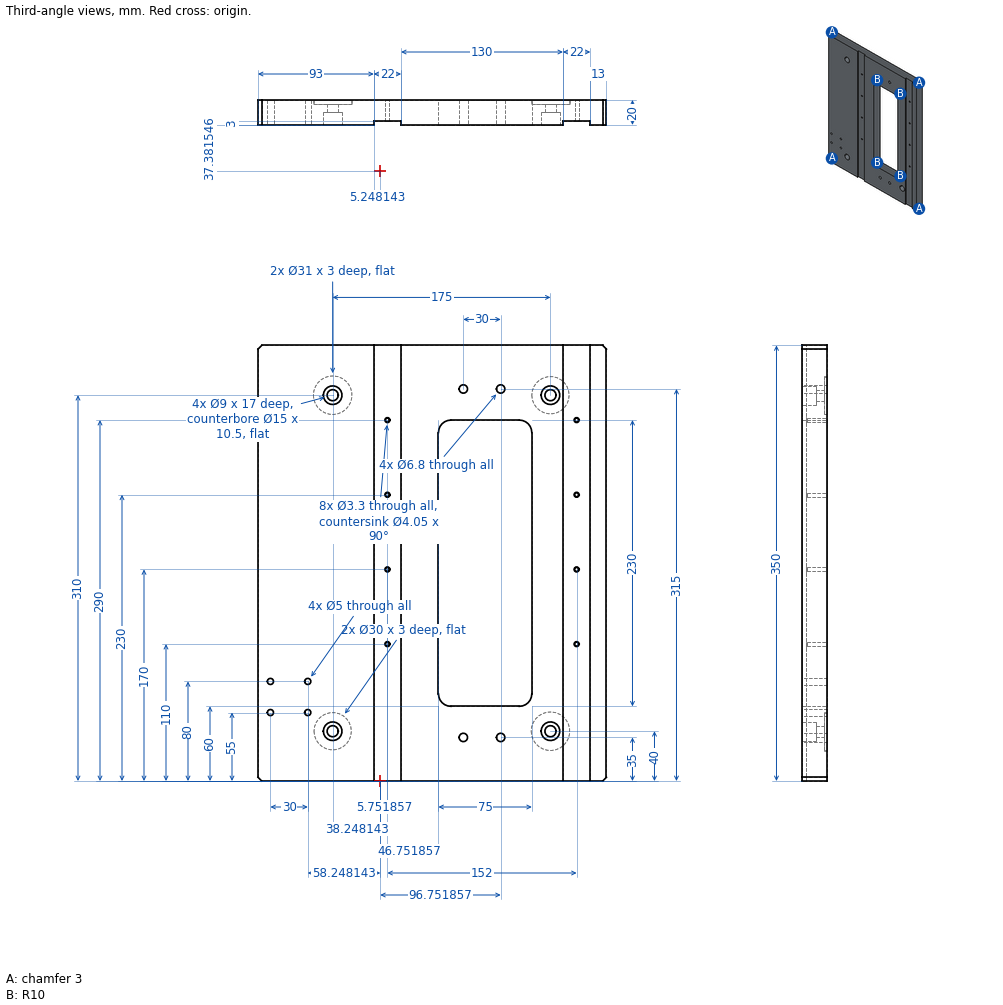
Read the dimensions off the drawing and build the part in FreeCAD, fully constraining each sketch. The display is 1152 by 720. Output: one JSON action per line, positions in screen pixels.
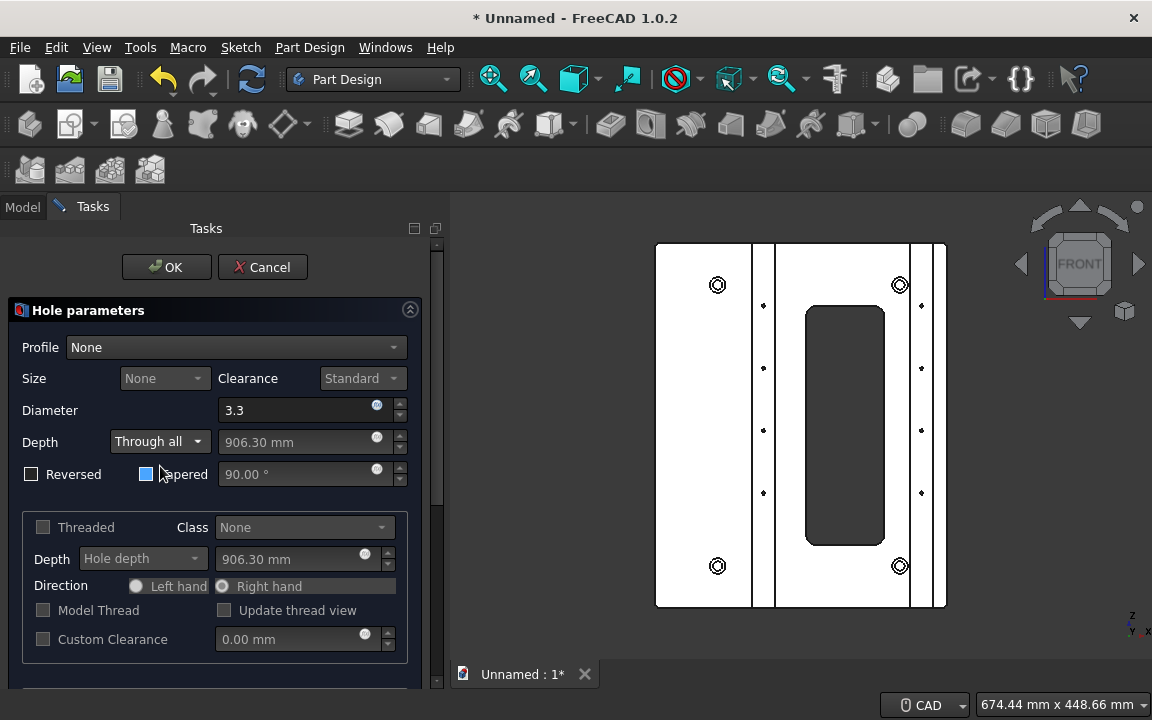
{"action": "scroll", "coordinate": [437, 463], "scroll_direction": "down", "scroll_amount": 2}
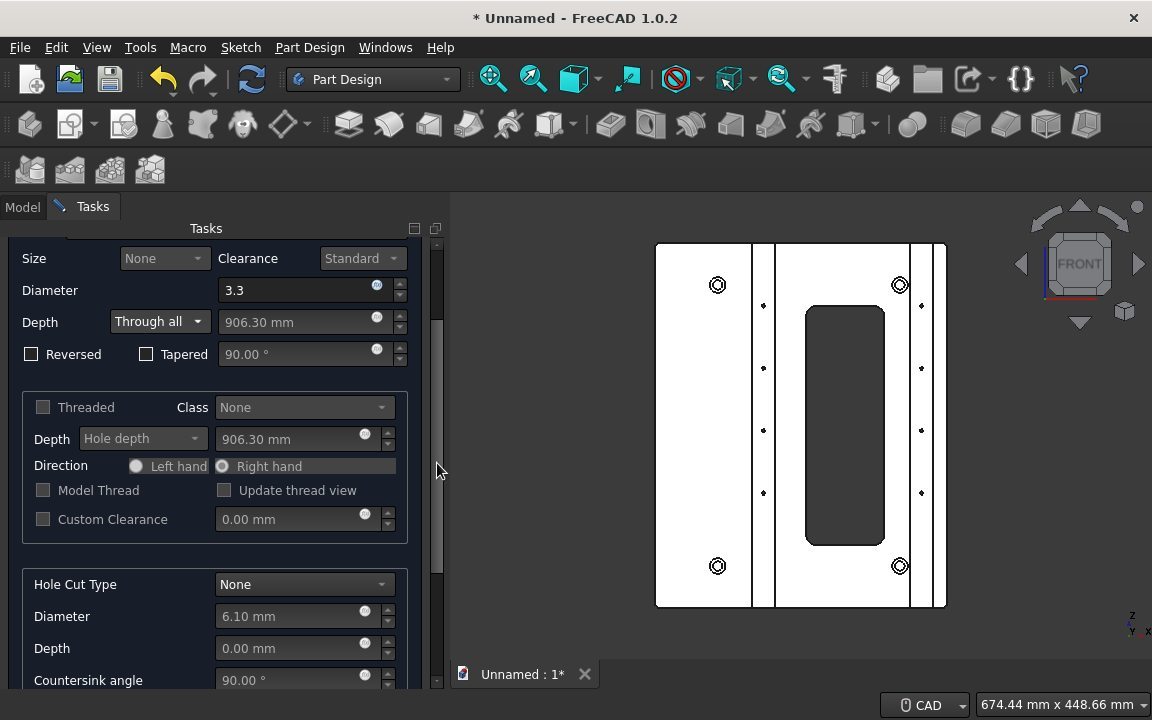
{"action": "left_click", "coordinate": [306, 584]}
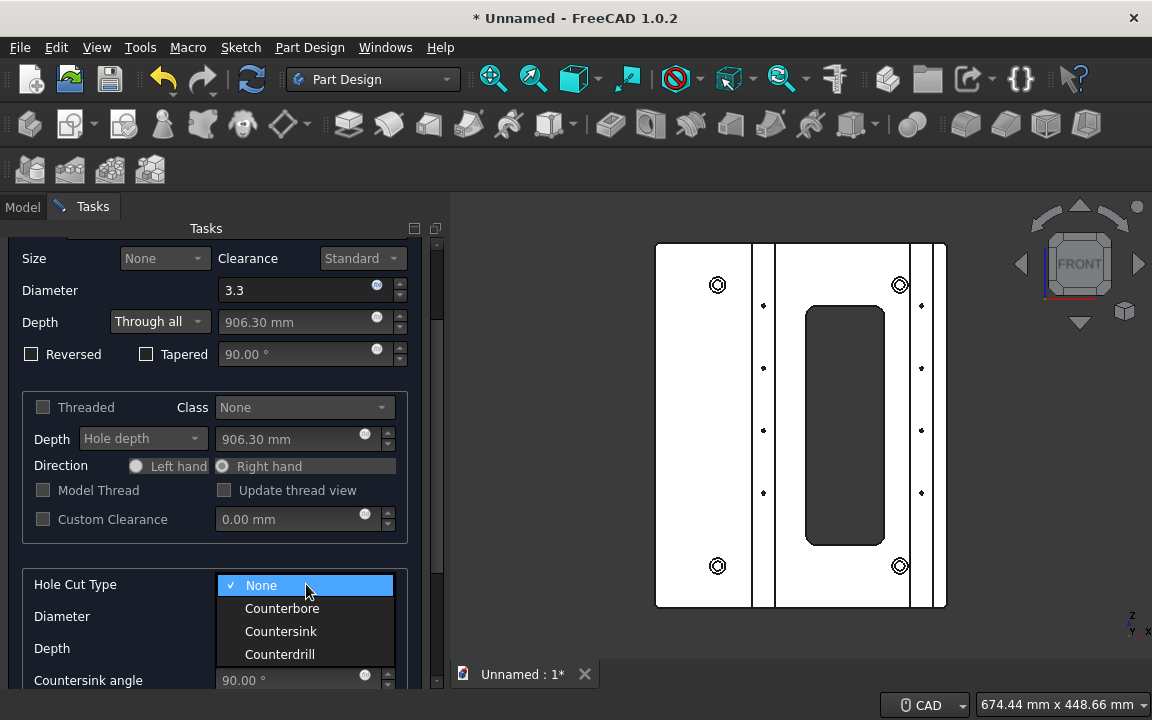
{"action": "left_click", "coordinate": [304, 632]}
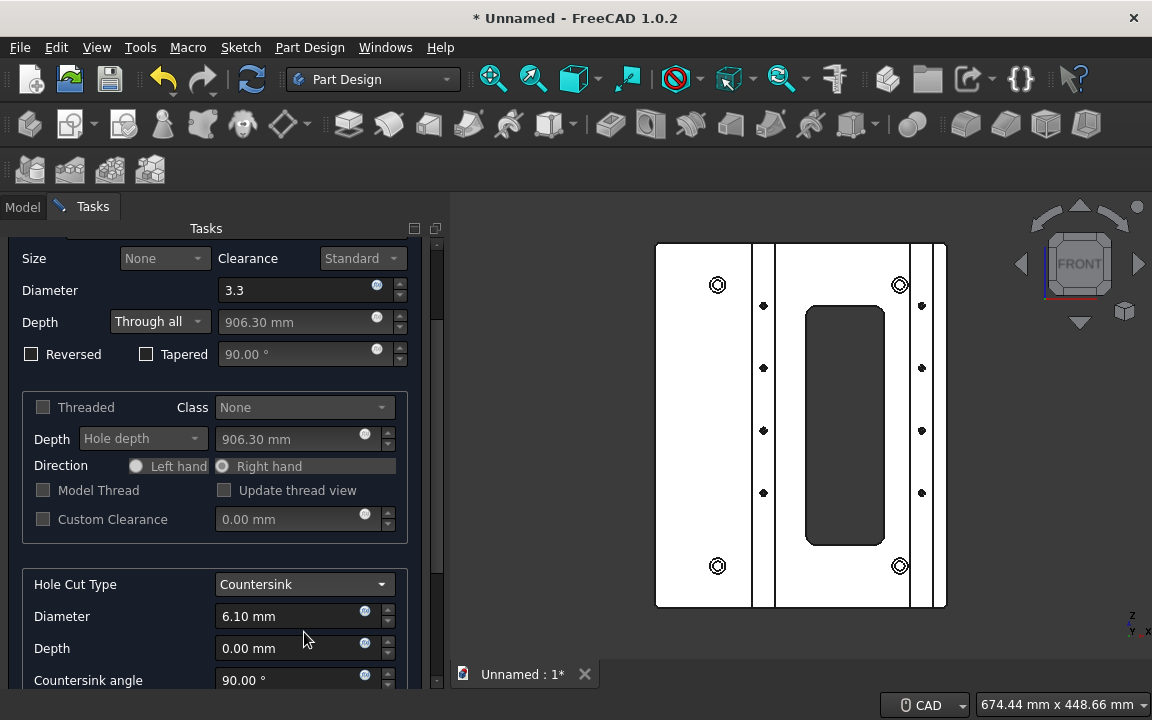
{"action": "triple_click", "coordinate": [298, 616]}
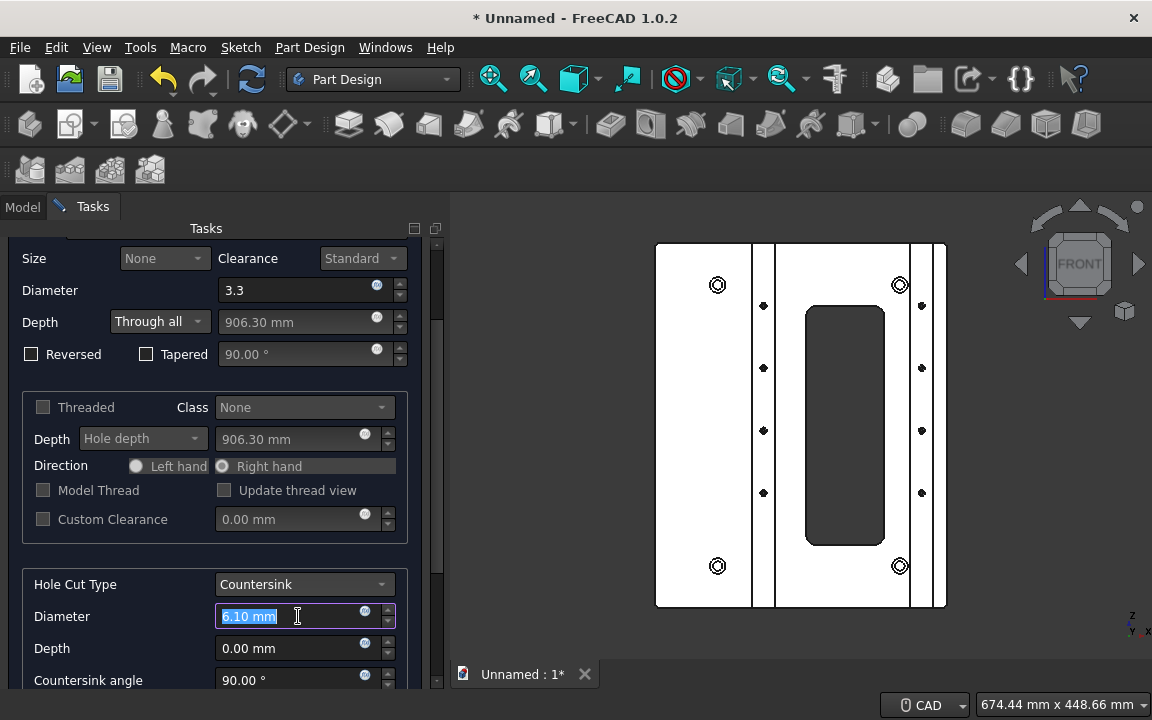
{"action": "type", "text": "4.05"}
{"action": "key", "text": "Tab"}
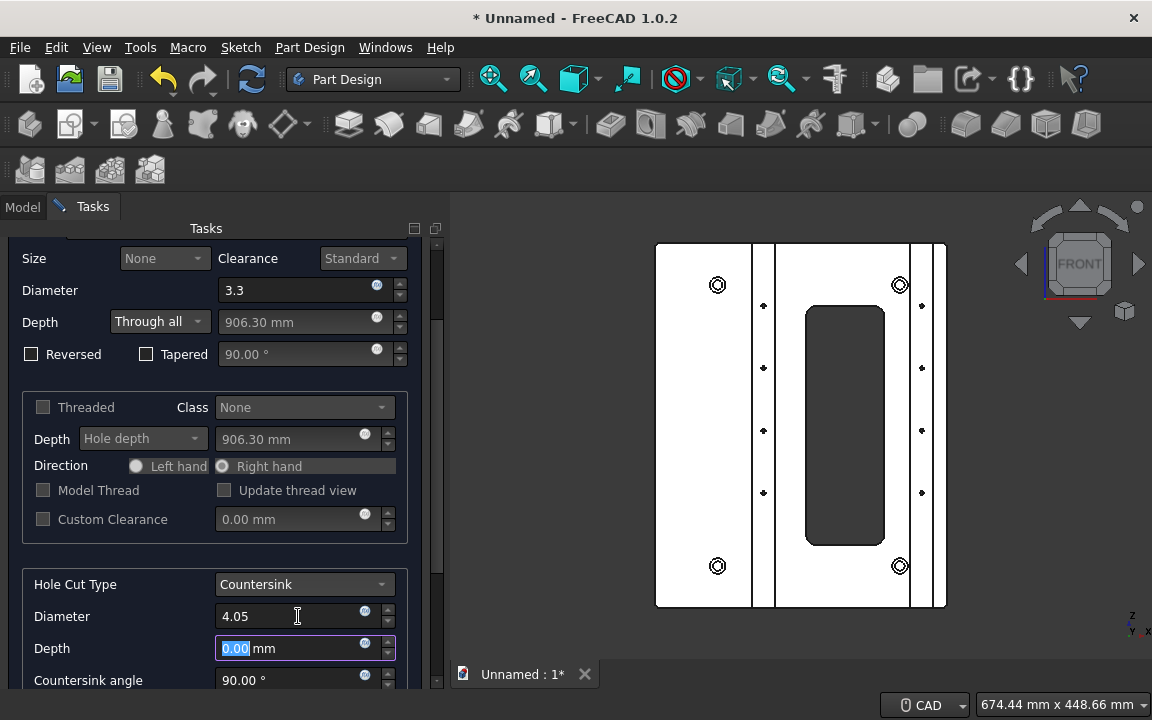
{"action": "scroll", "coordinate": [437, 463], "scroll_direction": "up", "scroll_amount": 3}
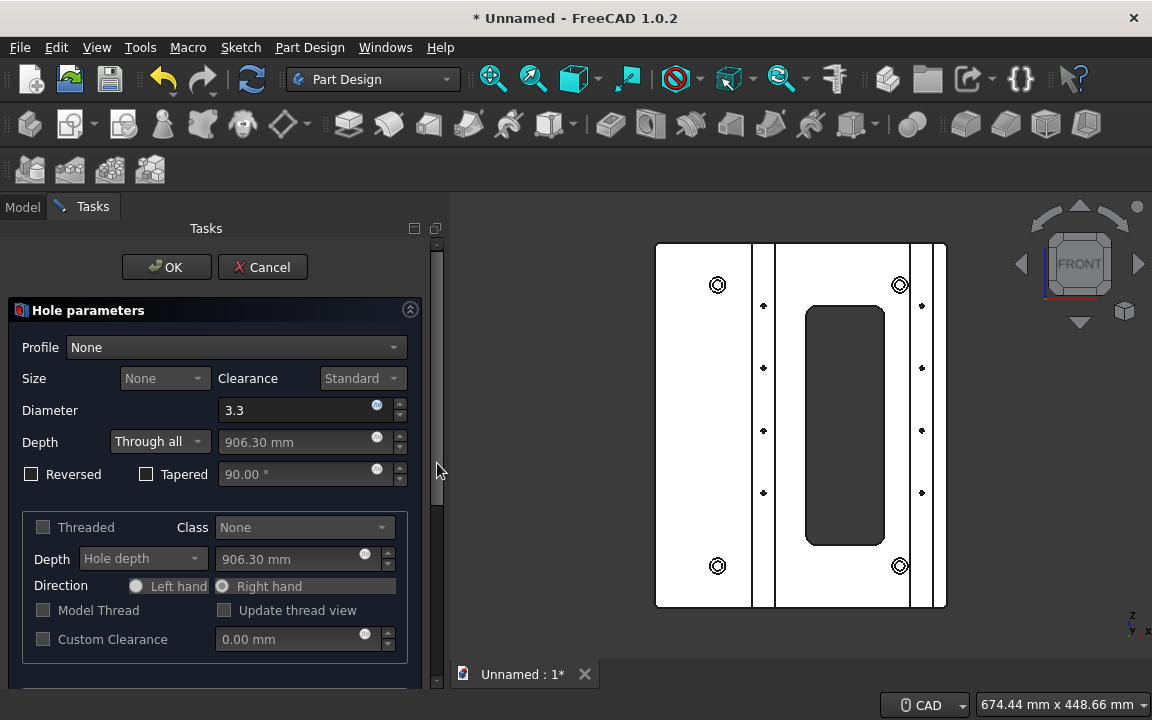
{"action": "left_click", "coordinate": [167, 267]}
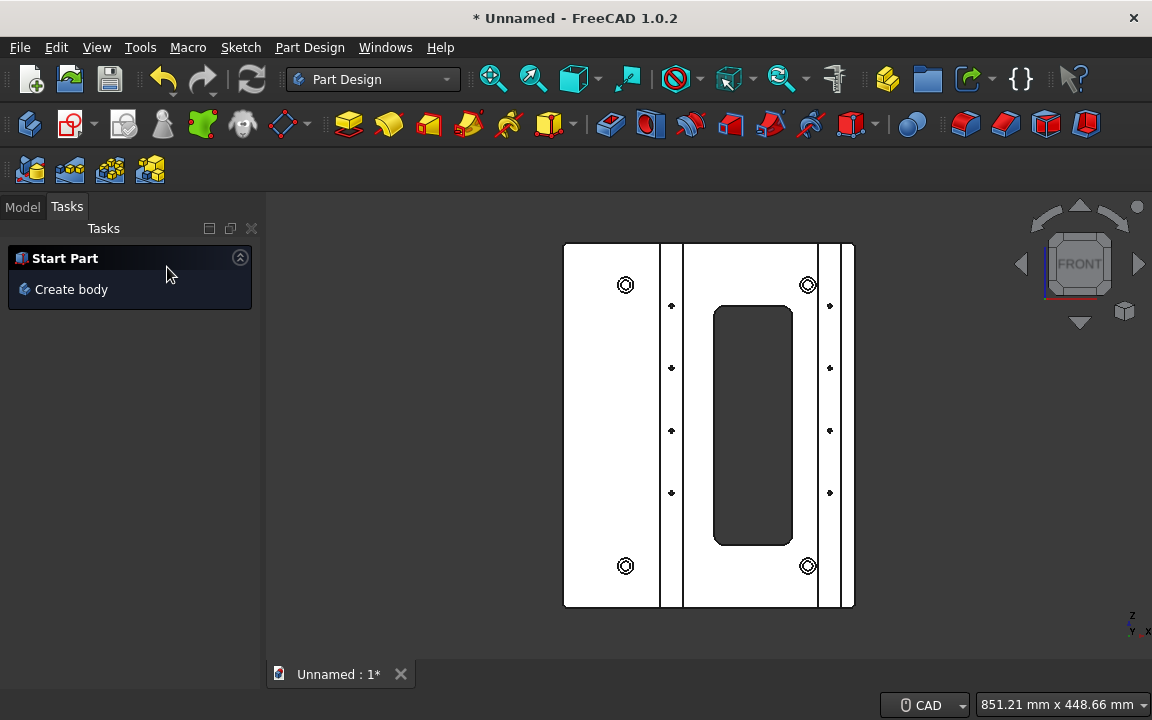
{"action": "key", "text": "4"}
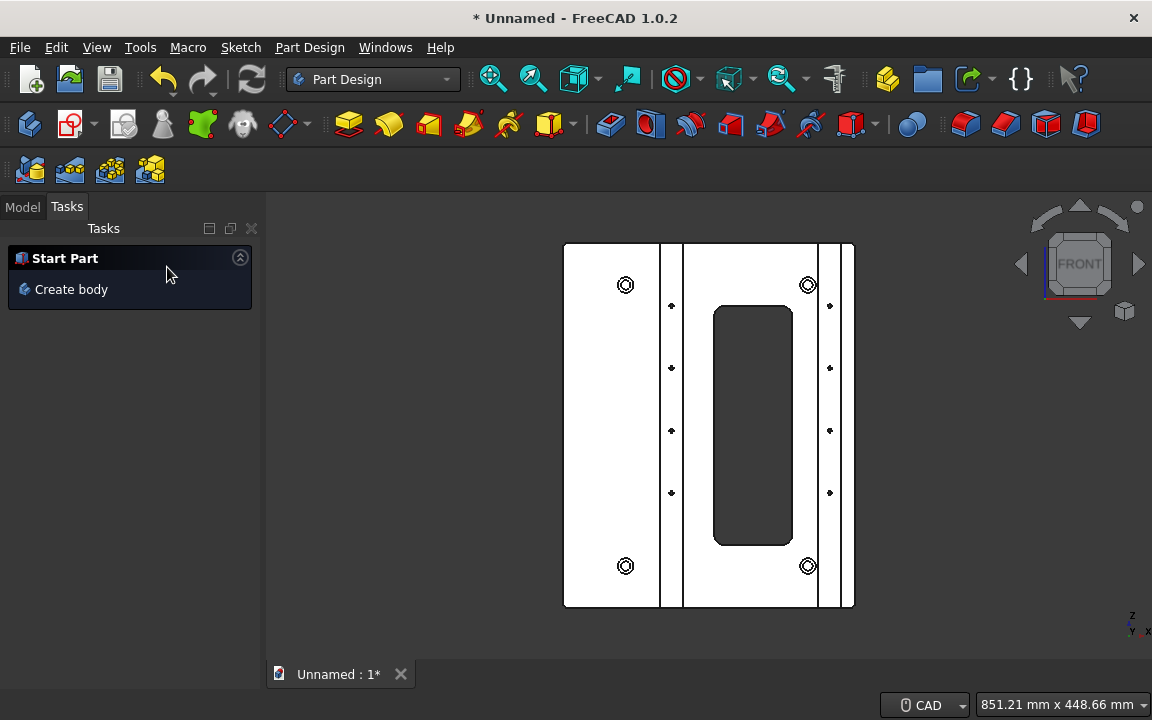
{"action": "left_click", "coordinate": [792, 529]}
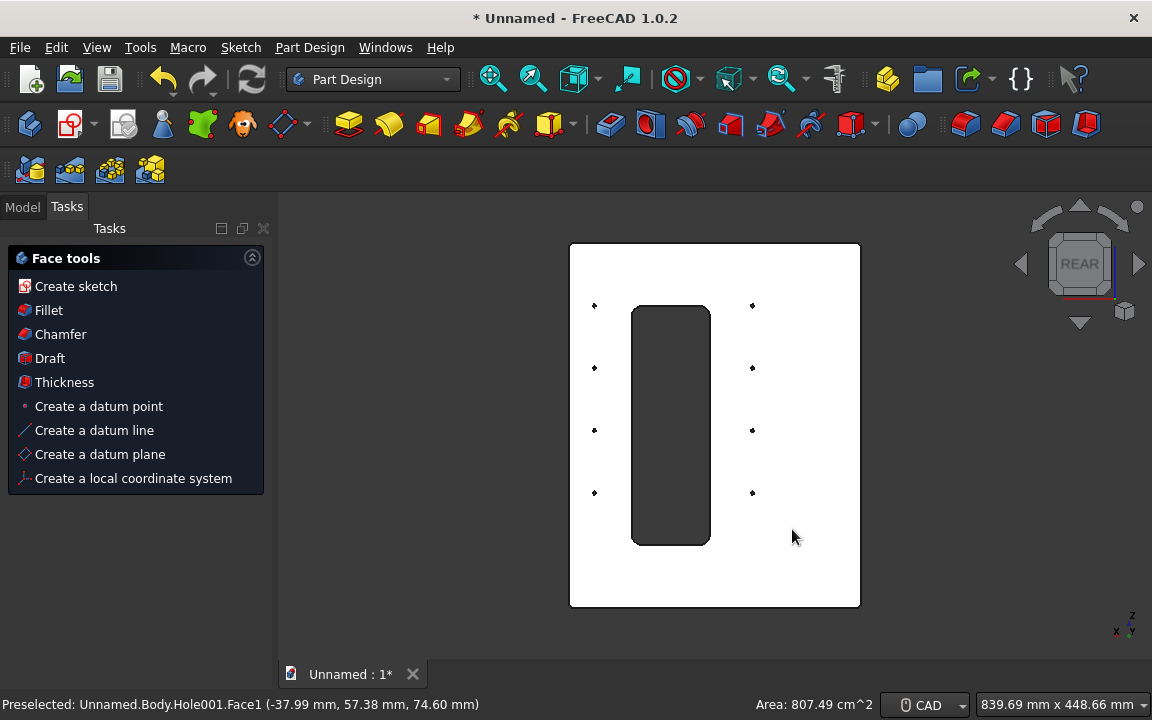
{"action": "left_click", "coordinate": [70, 124]}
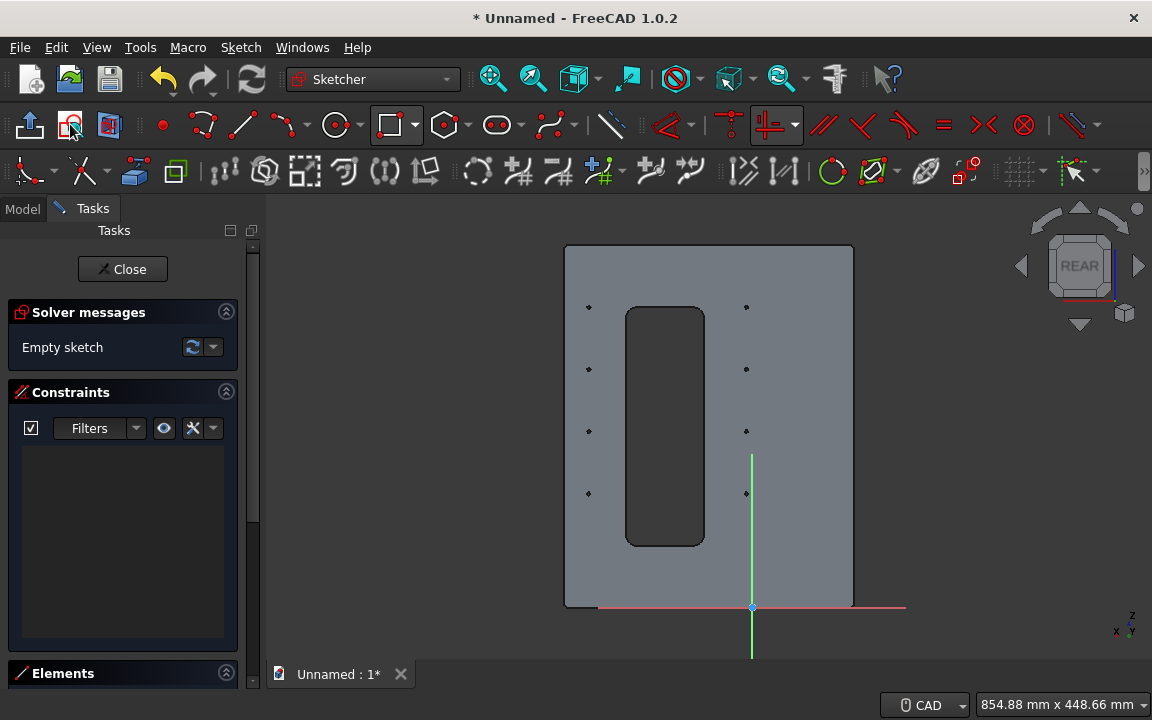
{"action": "scroll", "coordinate": [366, 369], "scroll_direction": "down", "scroll_amount": 1}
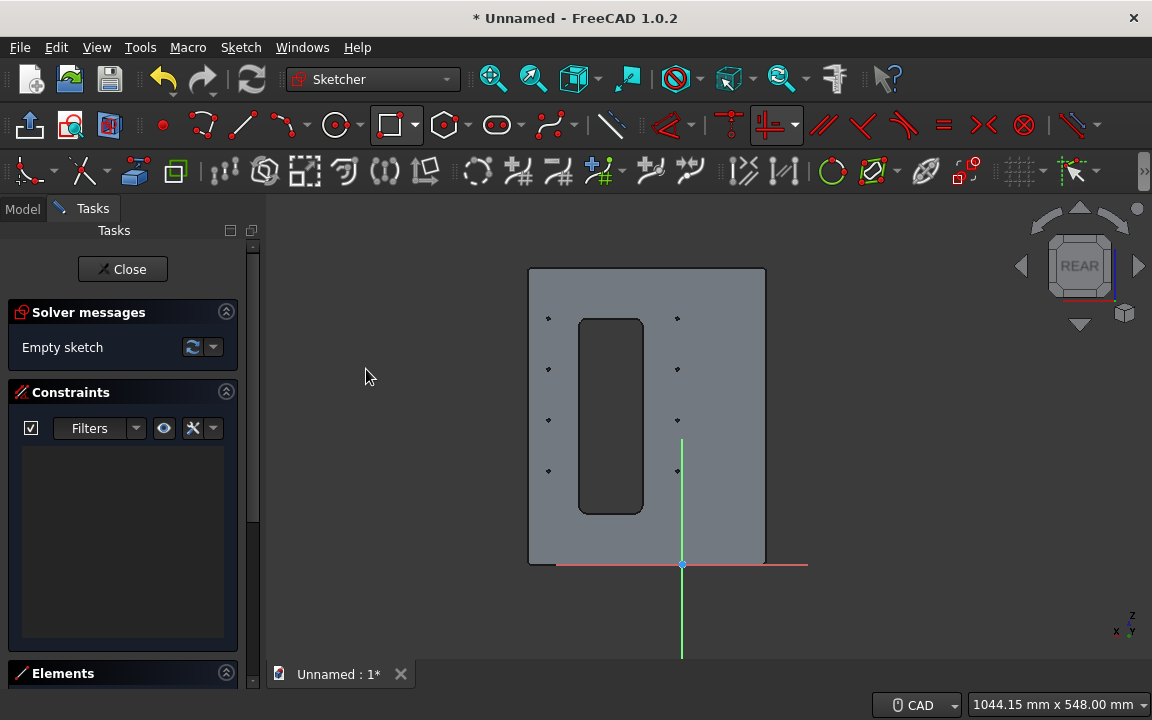
{"action": "left_click", "coordinate": [336, 126]}